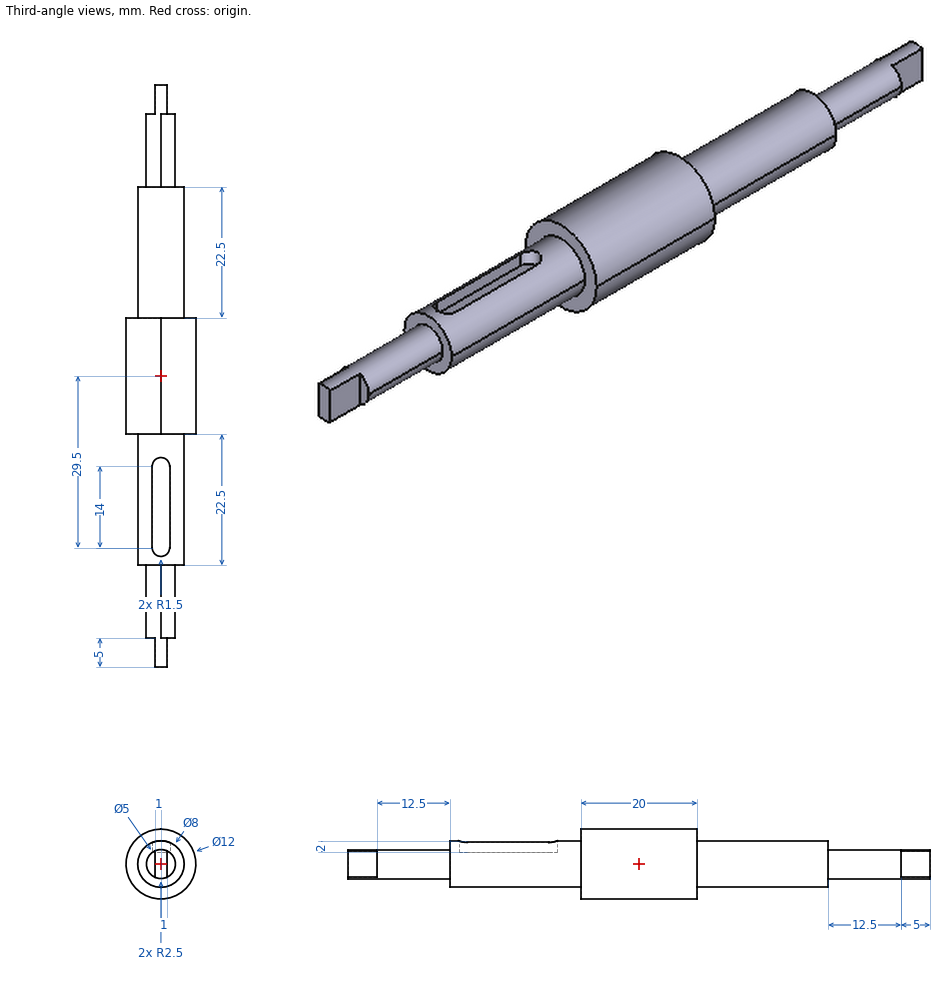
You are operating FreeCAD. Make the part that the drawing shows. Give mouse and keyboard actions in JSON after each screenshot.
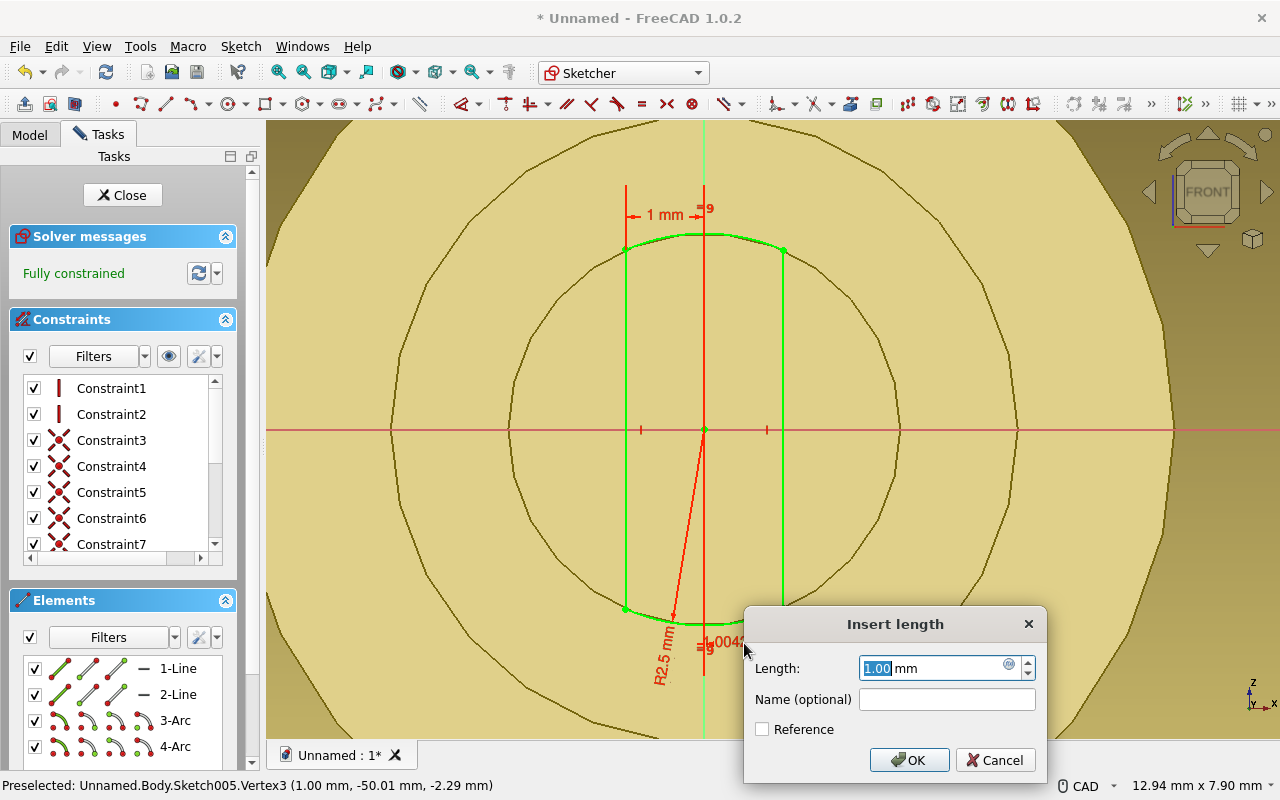
{"action": "type", "text": "1"}
{"action": "key", "text": "Return"}
{"action": "key", "text": "Escape"}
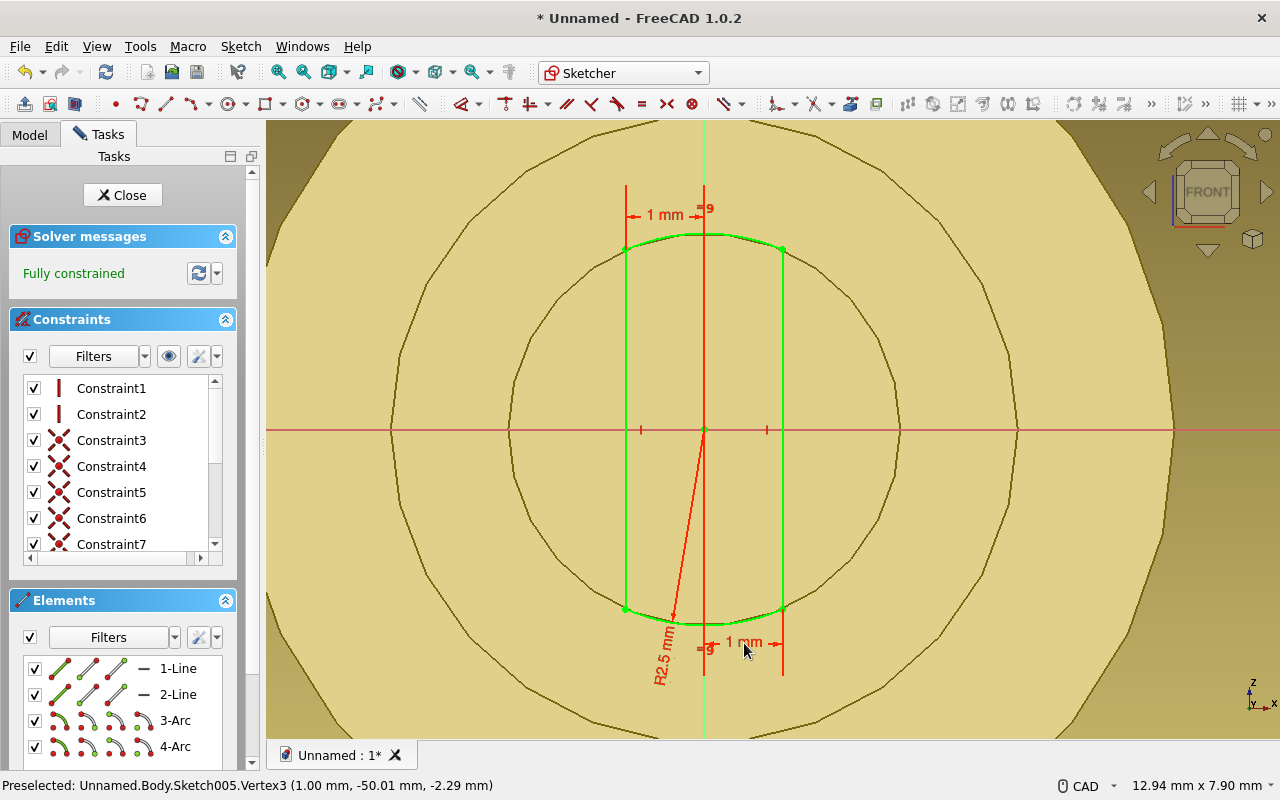
{"action": "left_click", "coordinate": [123, 195]}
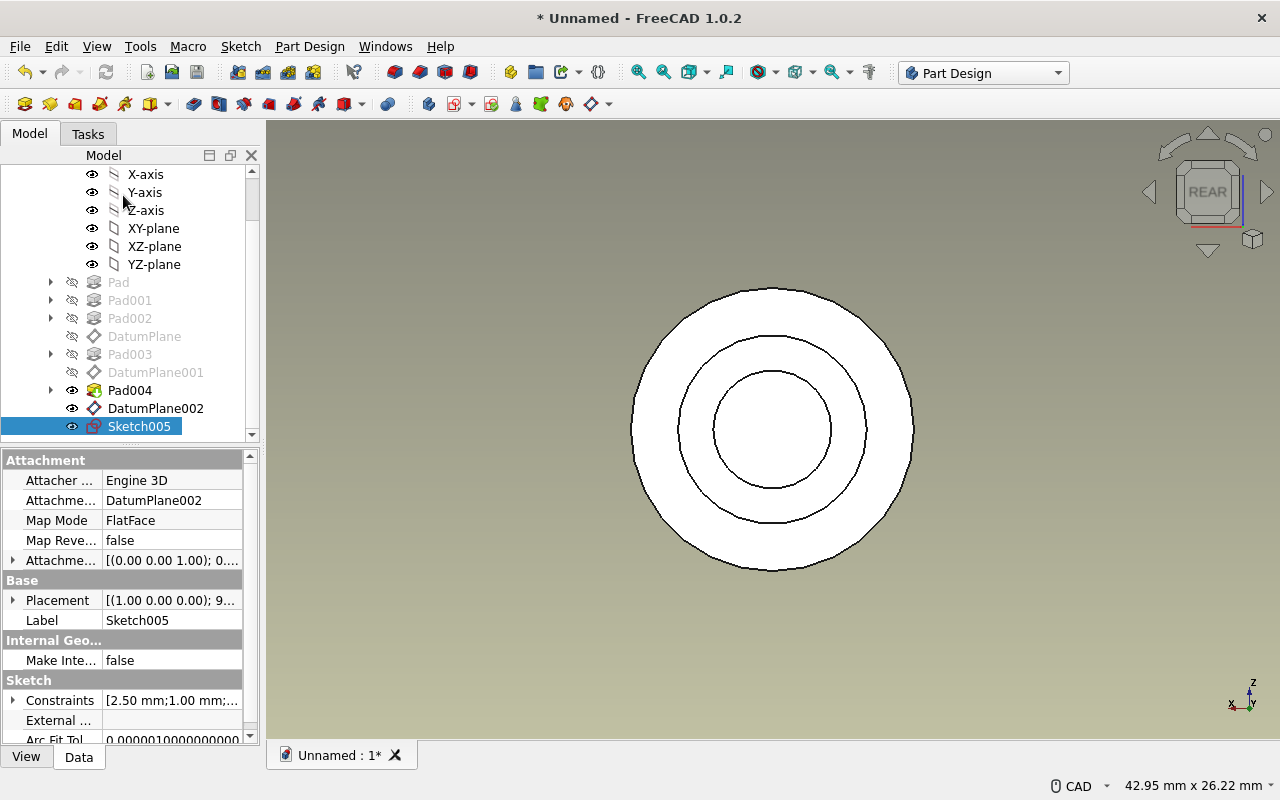
{"action": "left_click", "coordinate": [25, 104]}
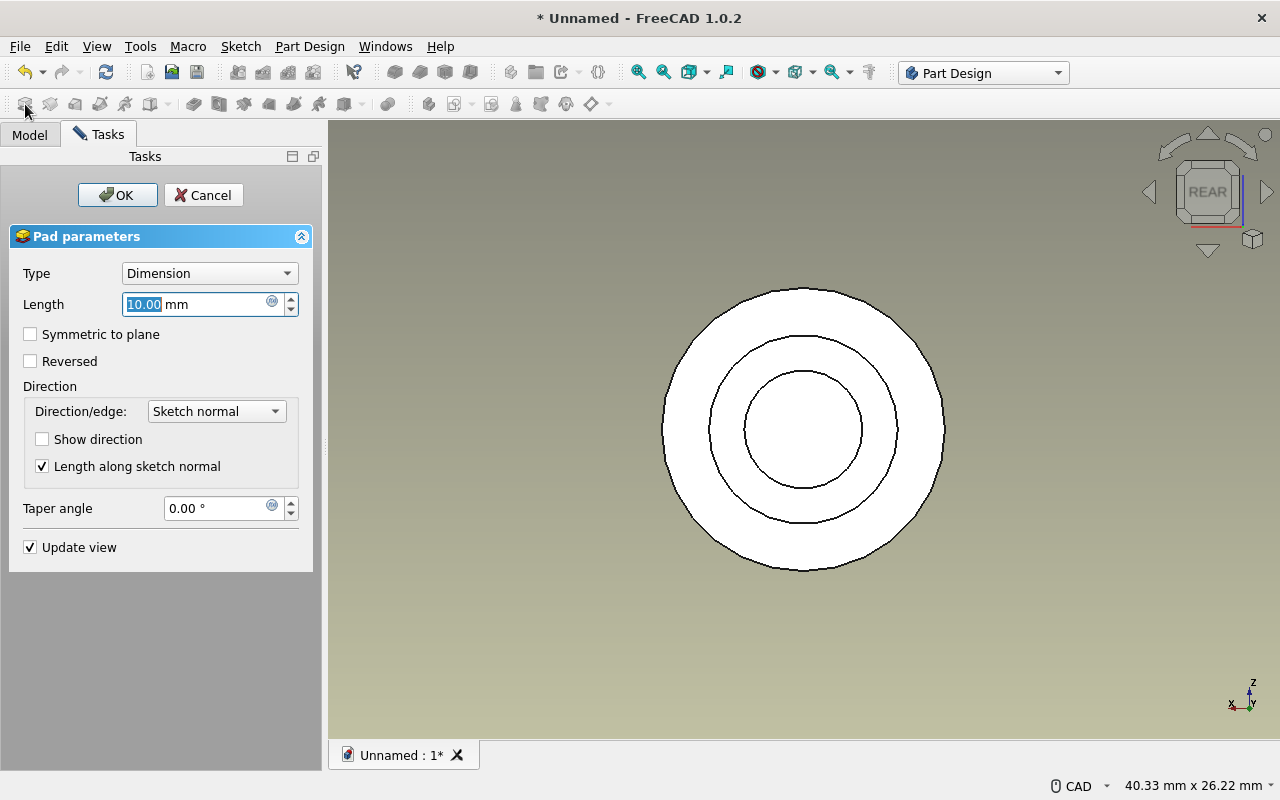
{"action": "type", "text": "5"}
{"action": "key", "text": "Tab"}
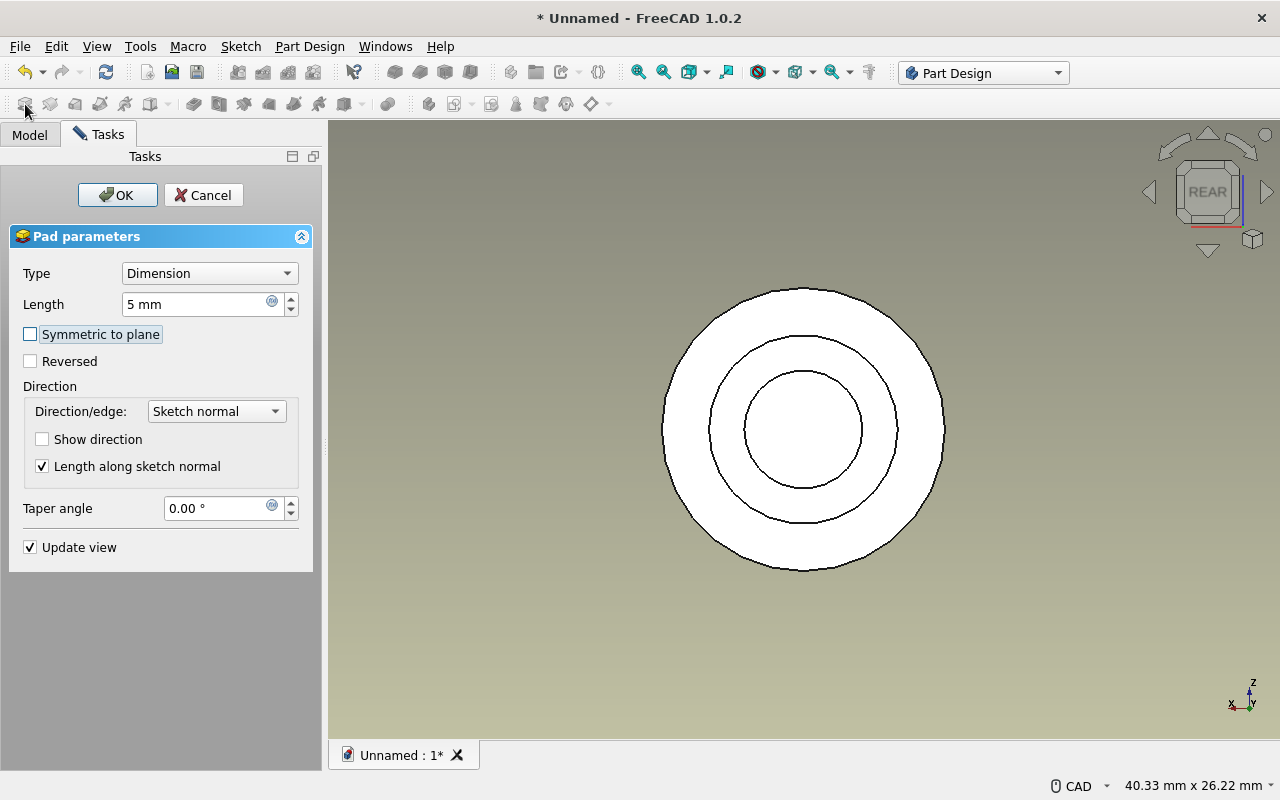
{"action": "left_click", "coordinate": [31, 361]}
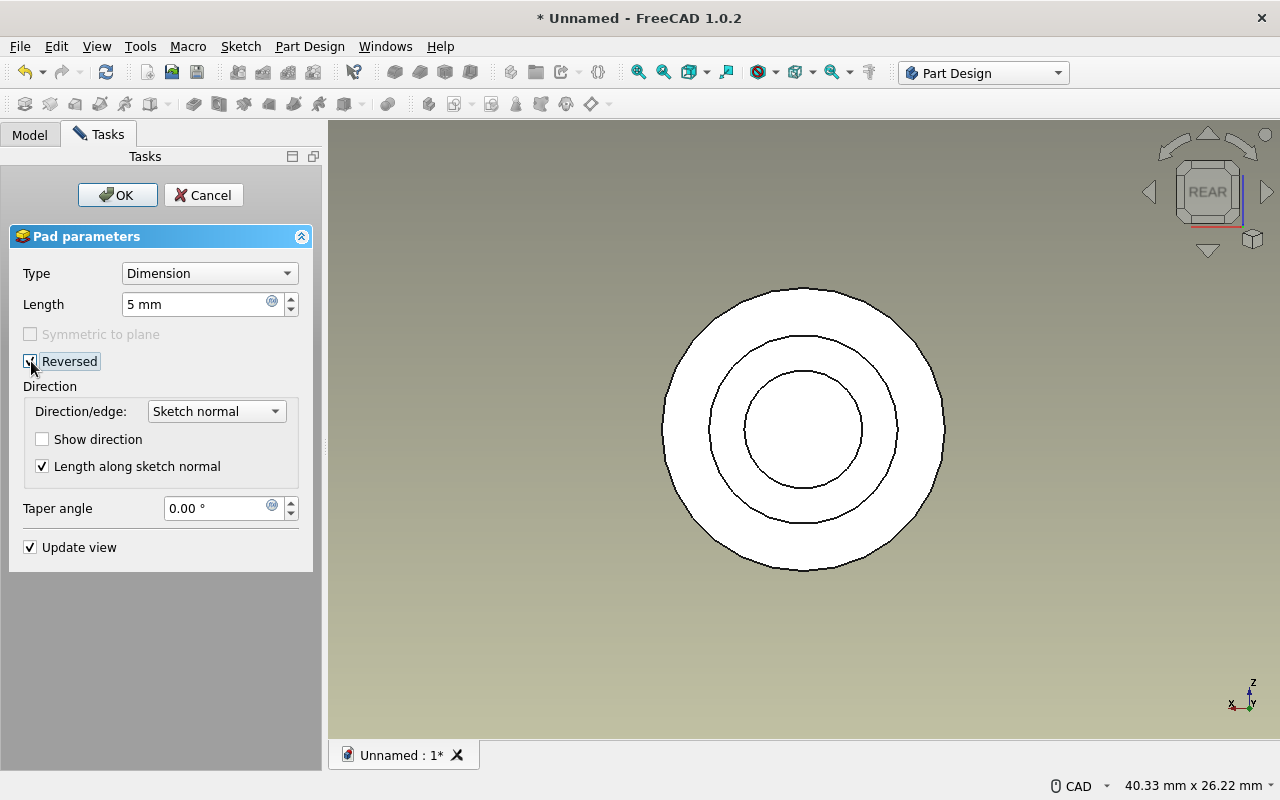
{"action": "left_click", "coordinate": [118, 195]}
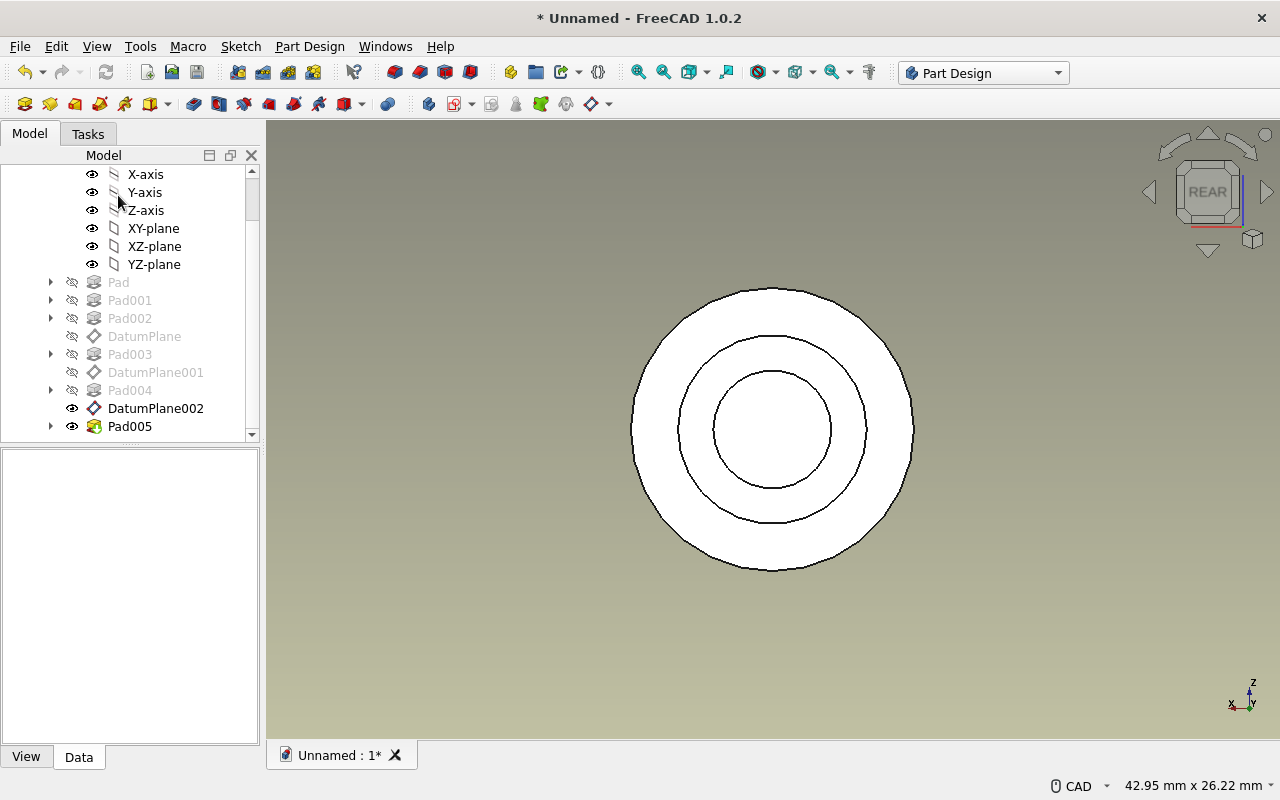
{"action": "left_click", "coordinate": [117, 408]}
{"action": "key", "text": "space"}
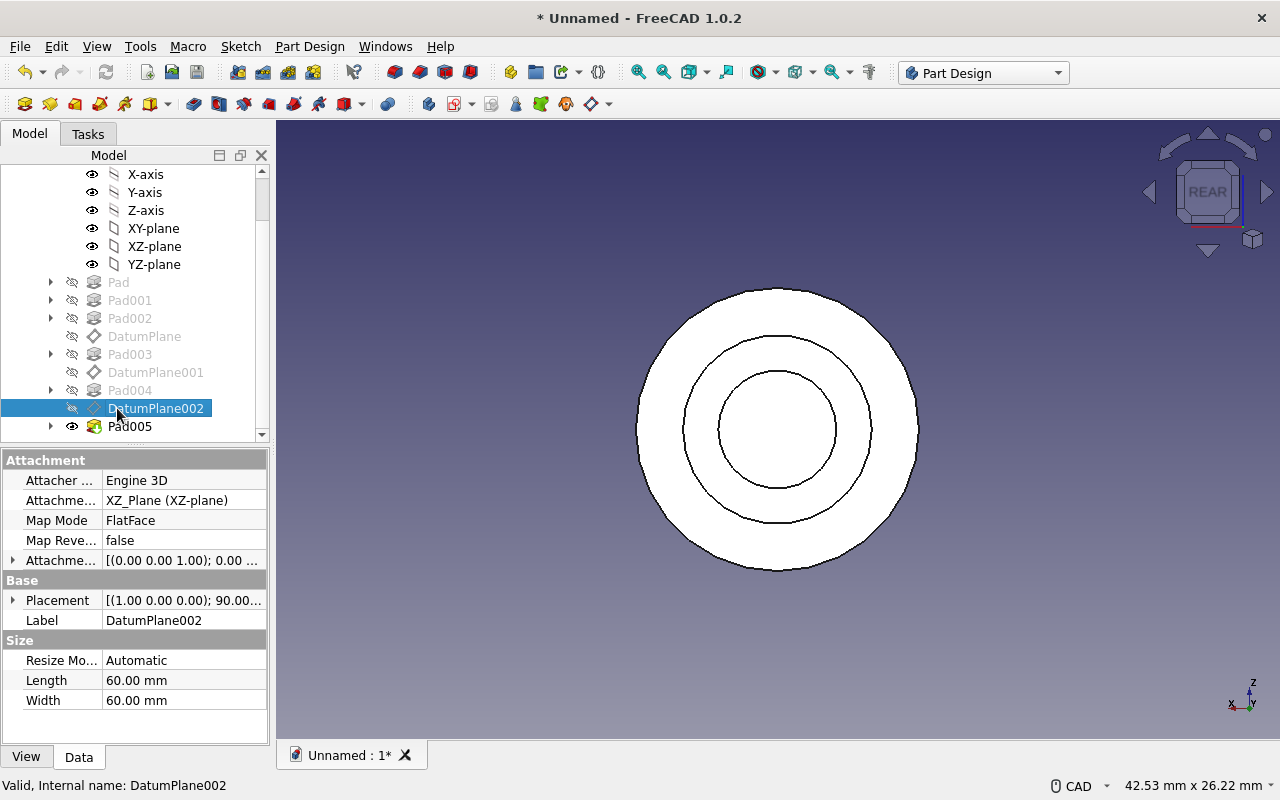
{"action": "left_click", "coordinate": [777, 428]}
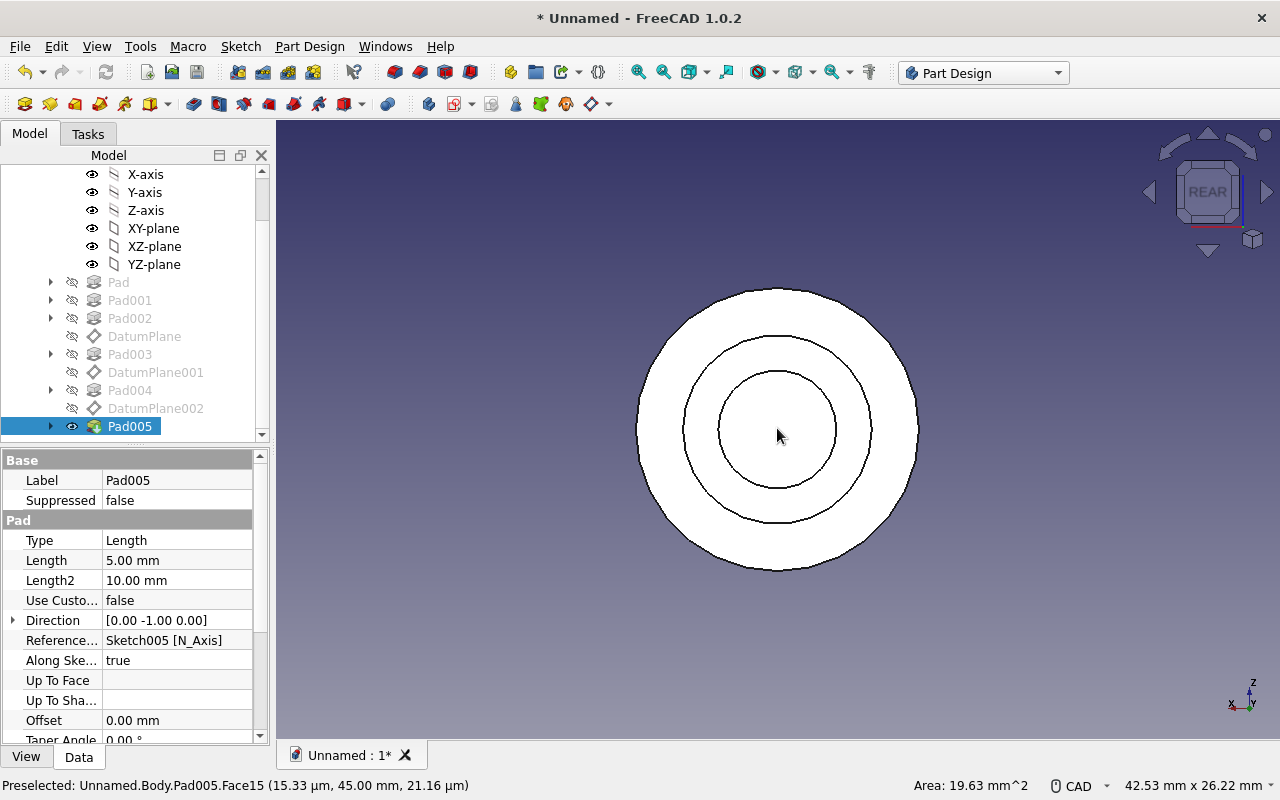
{"action": "left_click", "coordinate": [454, 104]}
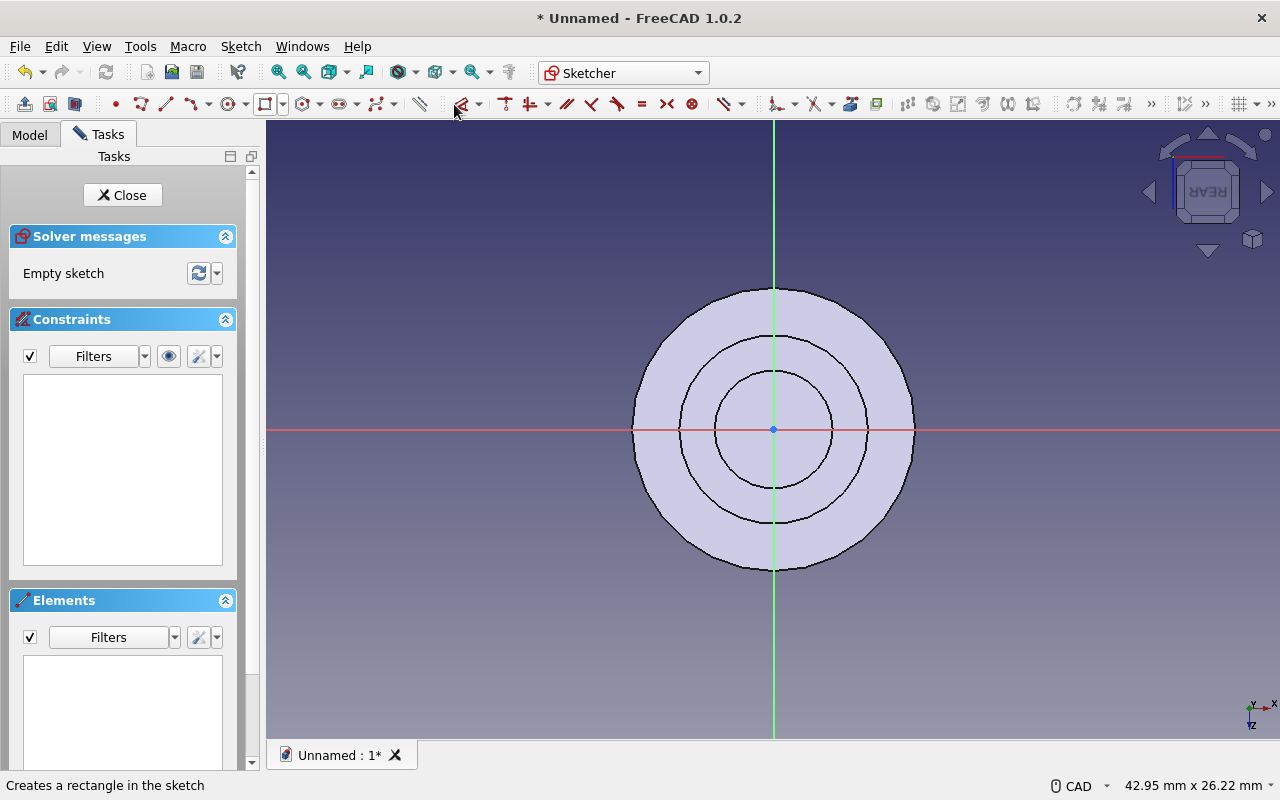
{"action": "scroll", "coordinate": [803, 430], "scroll_direction": "up", "scroll_amount": 6}